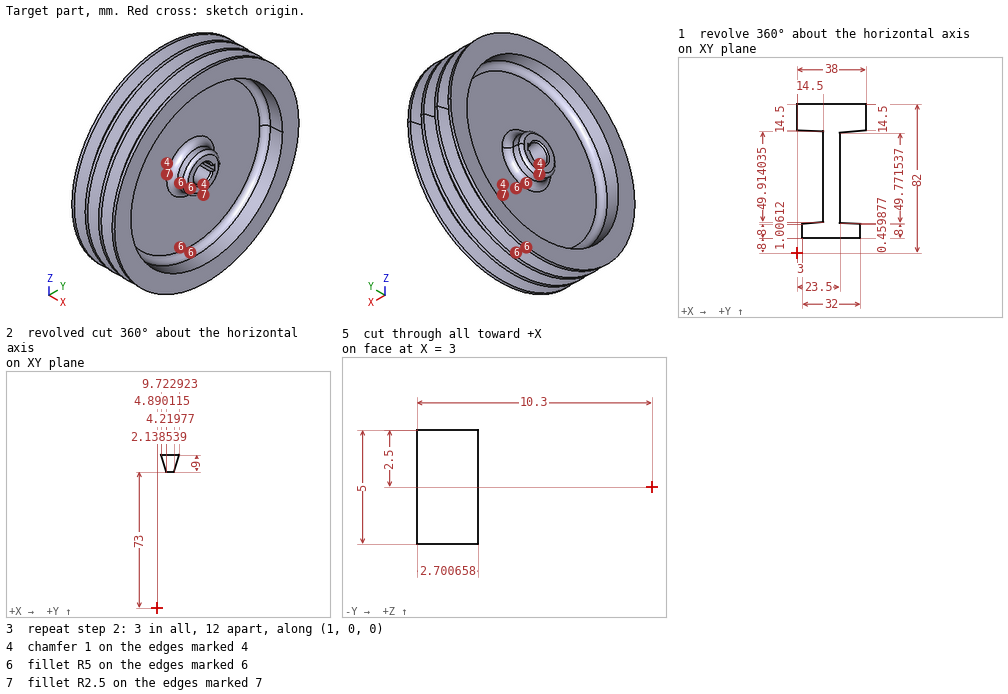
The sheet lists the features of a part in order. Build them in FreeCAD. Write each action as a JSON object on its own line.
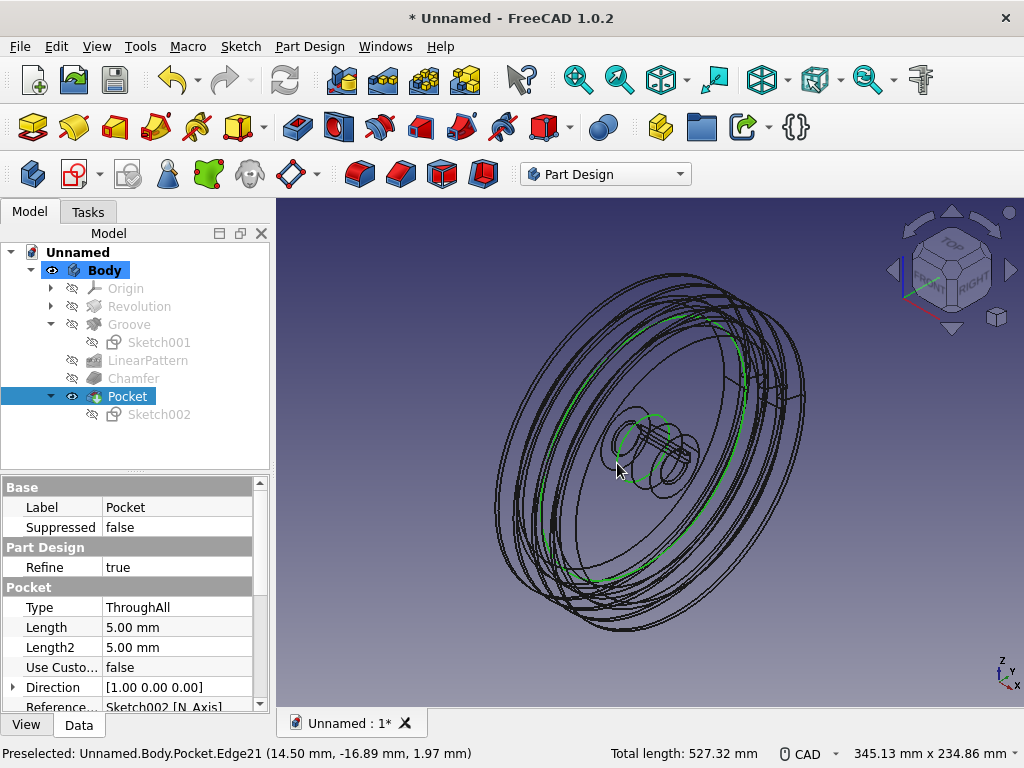
{"action": "left_click", "coordinate": [632, 470], "text": "ctrl"}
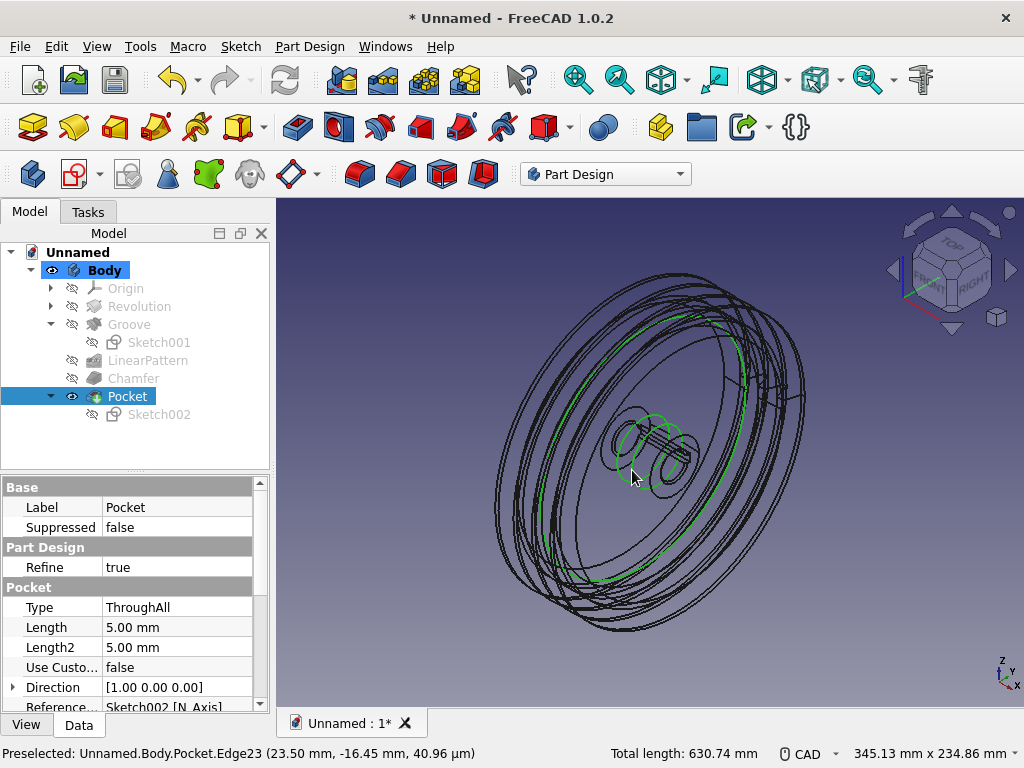
{"action": "left_click", "coordinate": [575, 572], "text": "ctrl"}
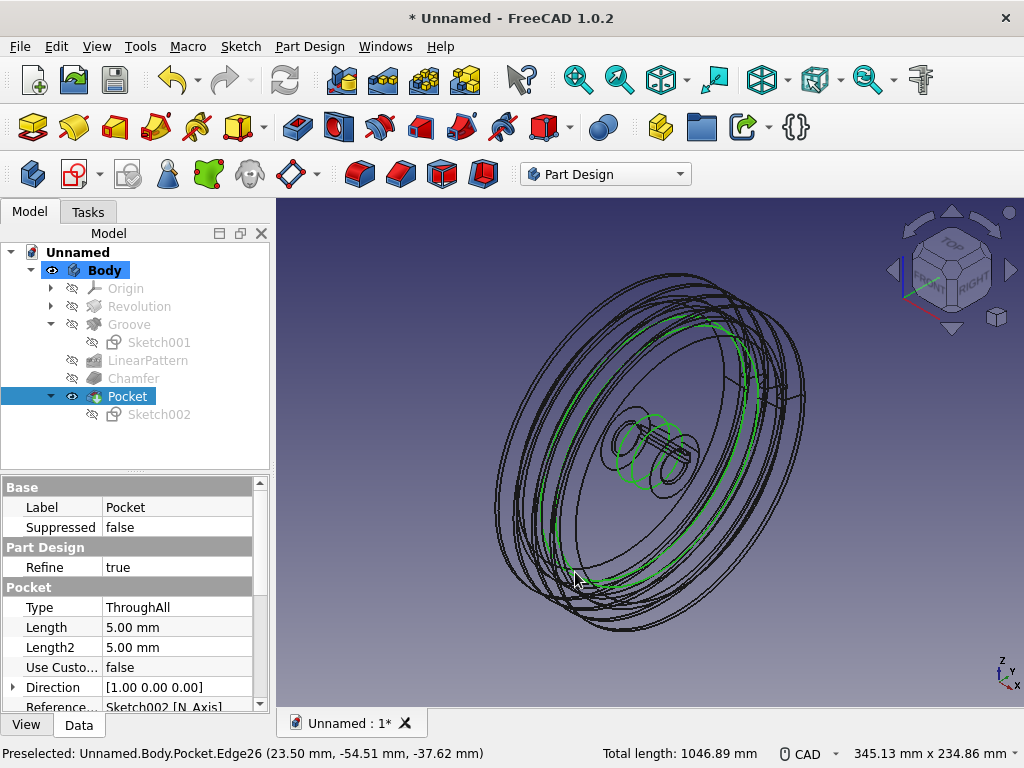
{"action": "key", "text": "v 1"}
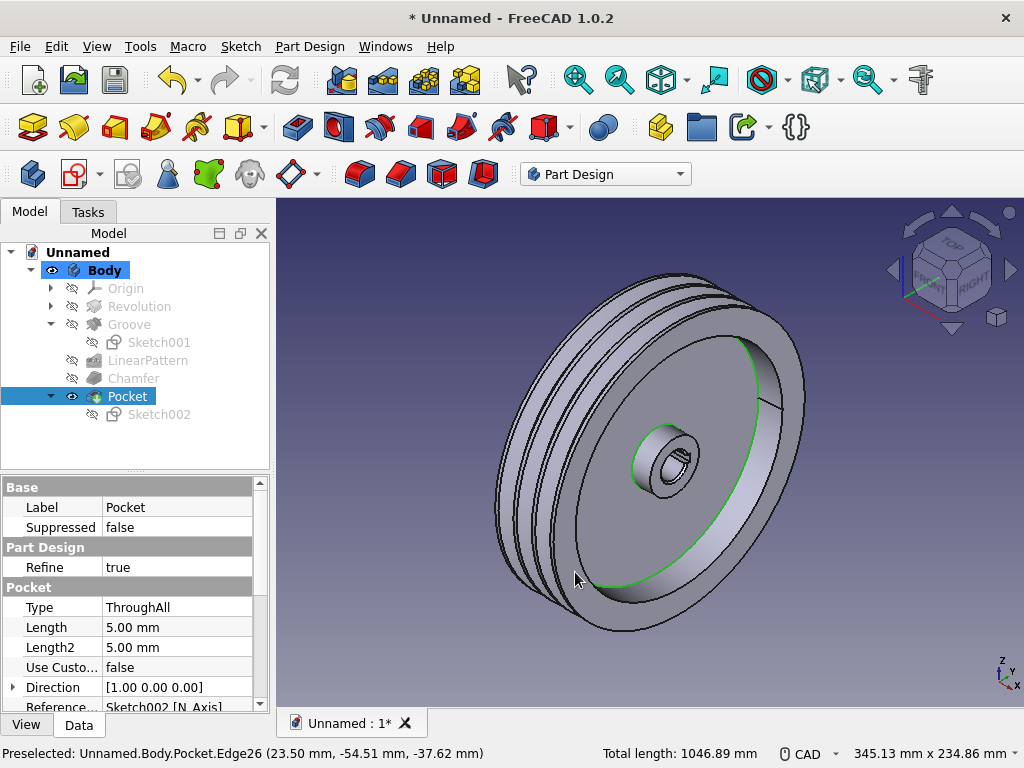
{"action": "left_click", "coordinate": [360, 174]}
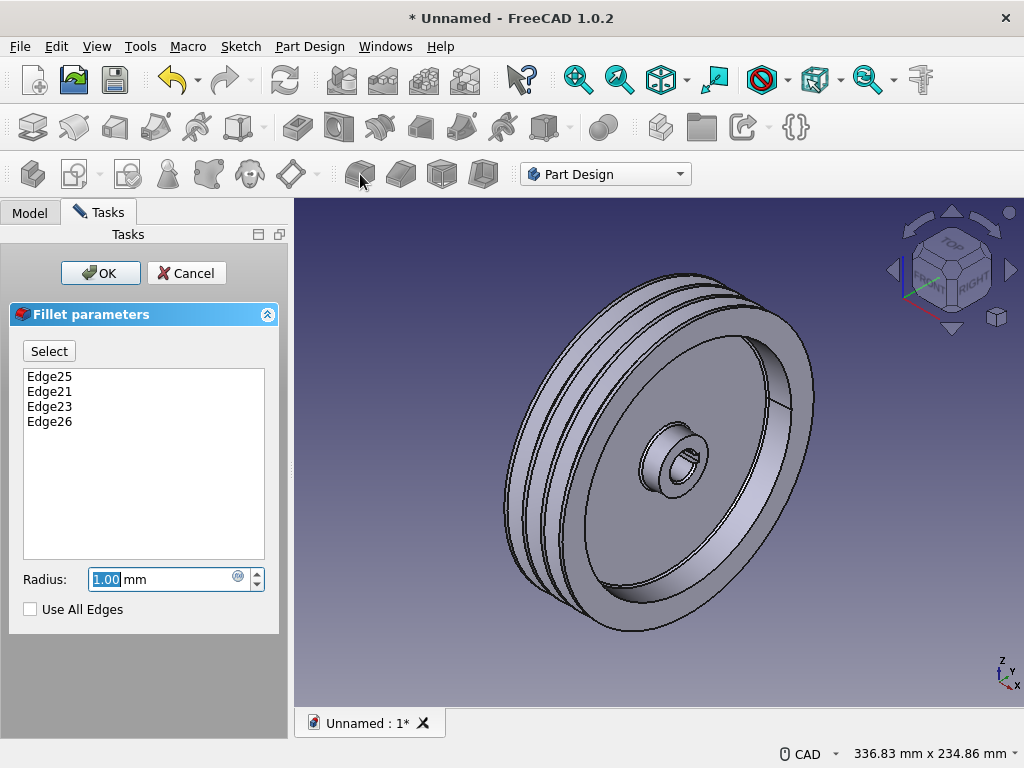
{"action": "type", "text": "5"}
{"action": "key", "text": "Tab"}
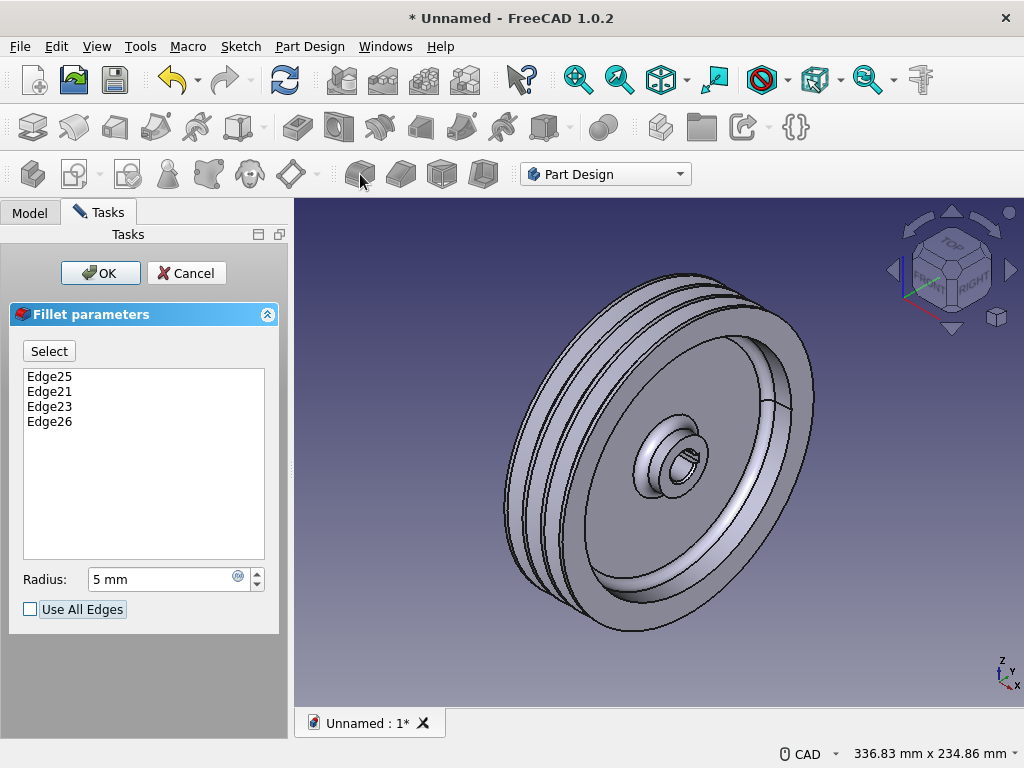
{"action": "left_click", "coordinate": [101, 273]}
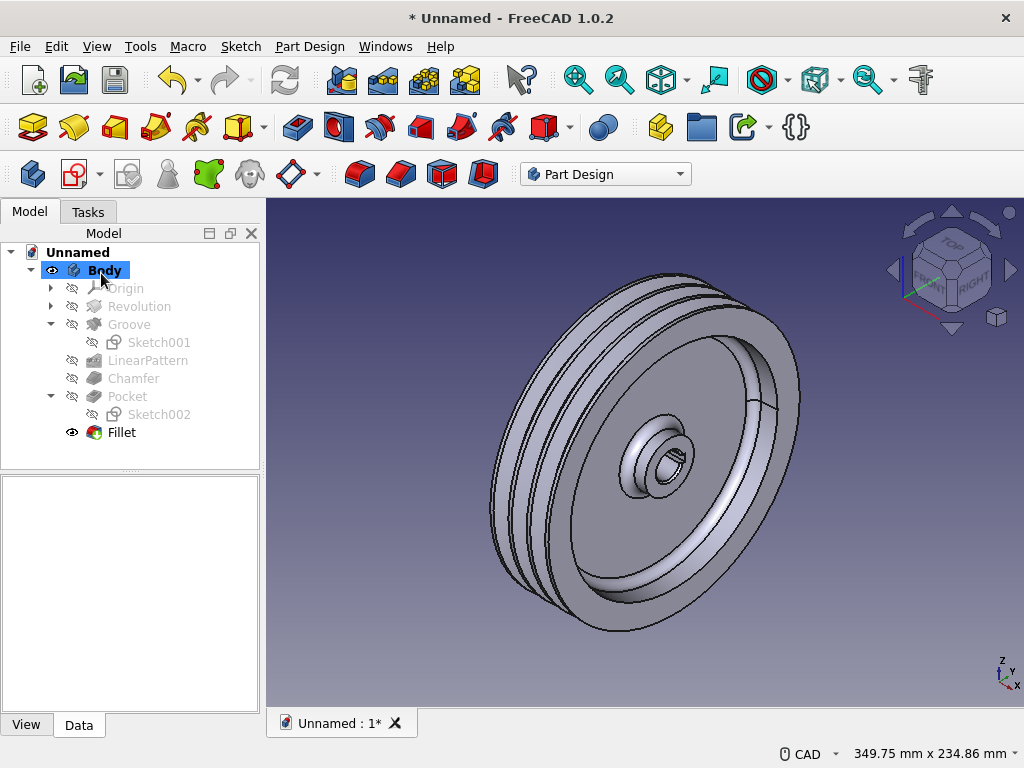
{"action": "left_click", "coordinate": [645, 480]}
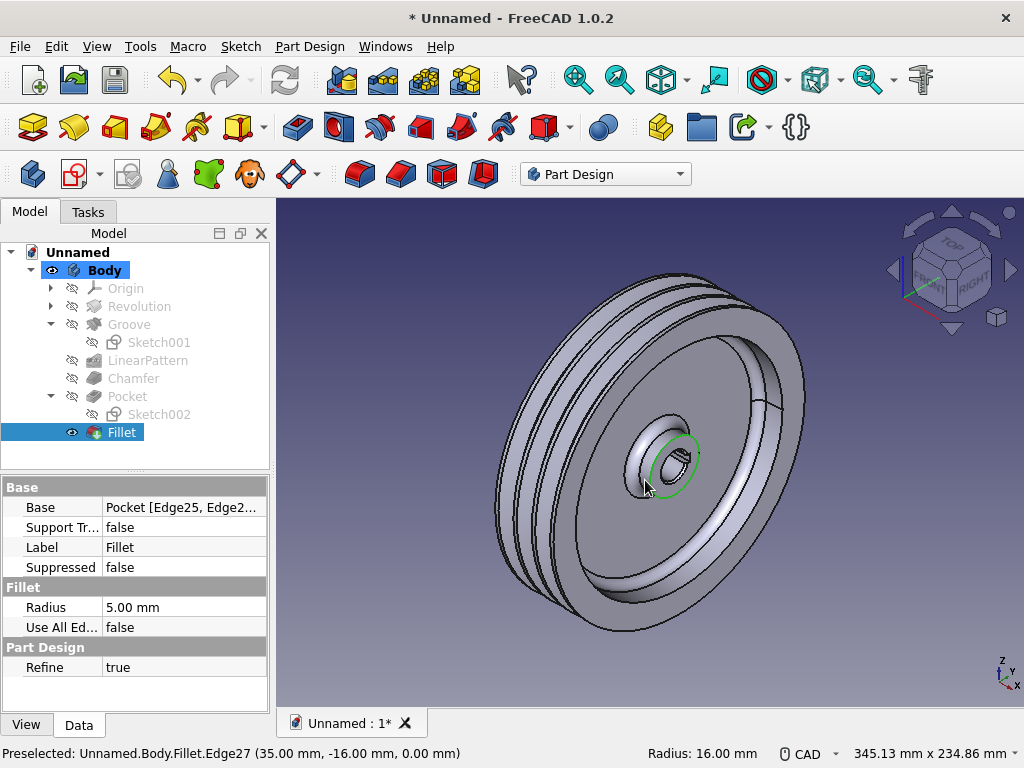
{"action": "key", "text": "2"}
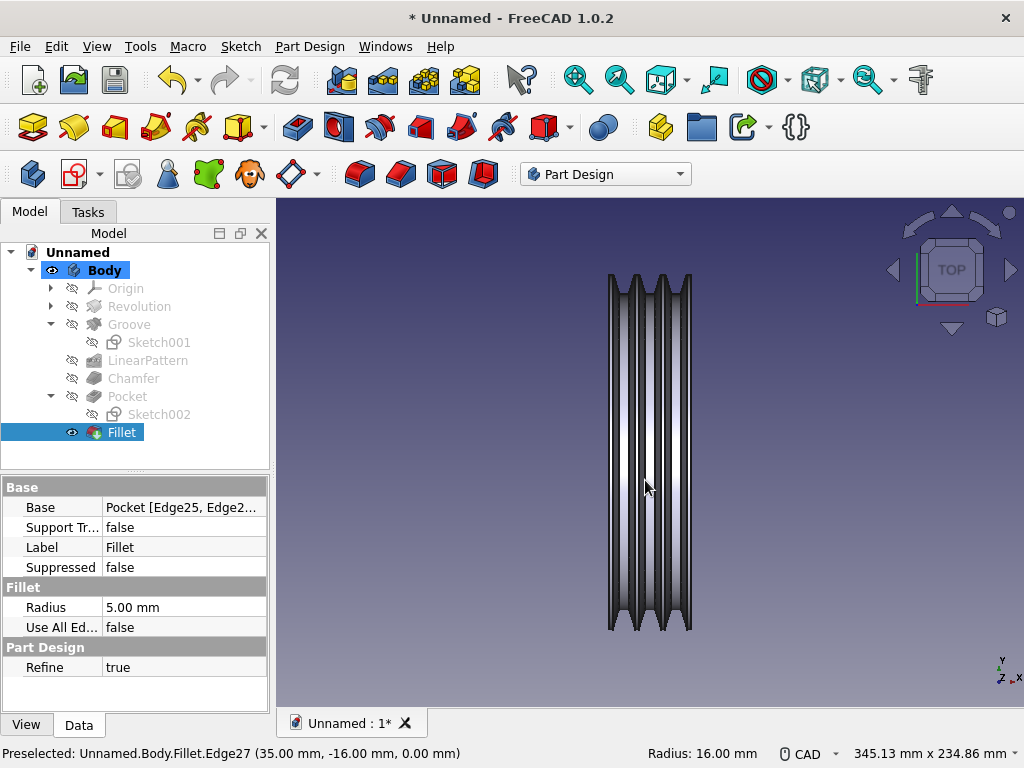
{"action": "key", "text": "0"}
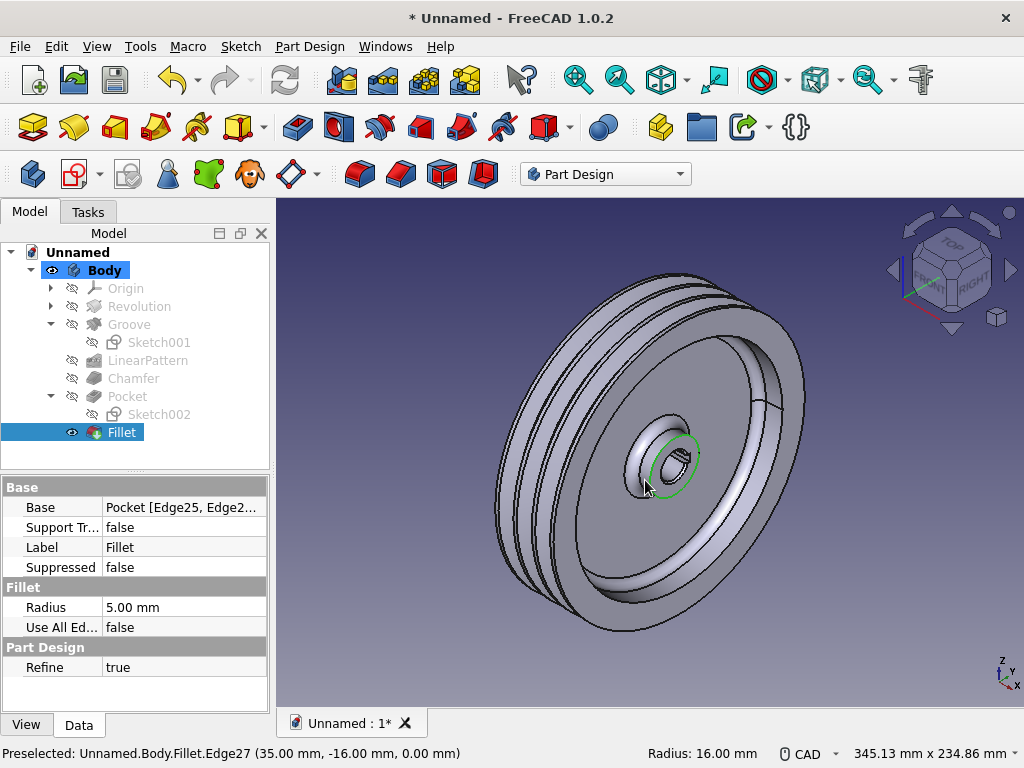
{"action": "key", "text": "1"}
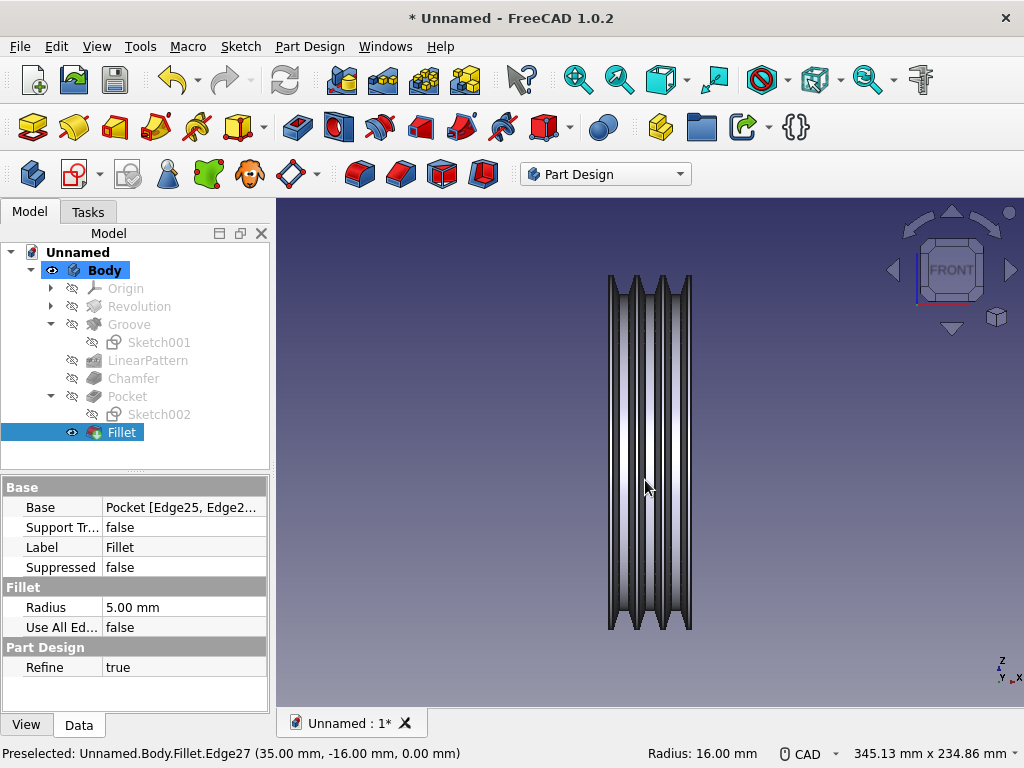
{"action": "key", "text": "3"}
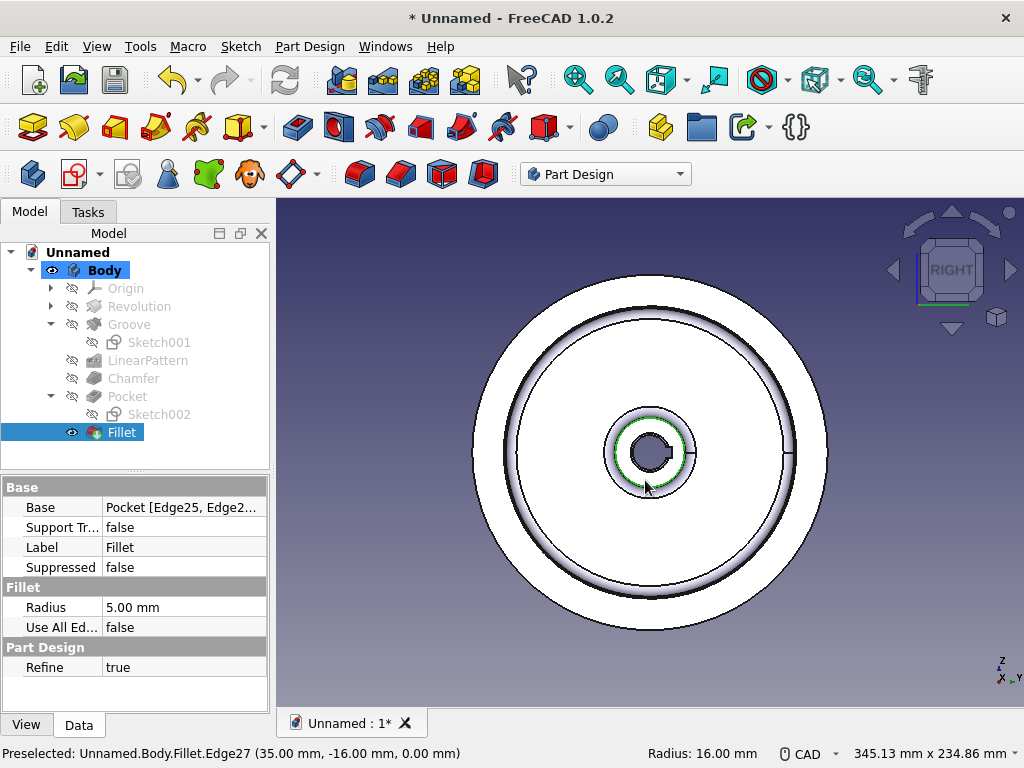
{"action": "key", "text": "5"}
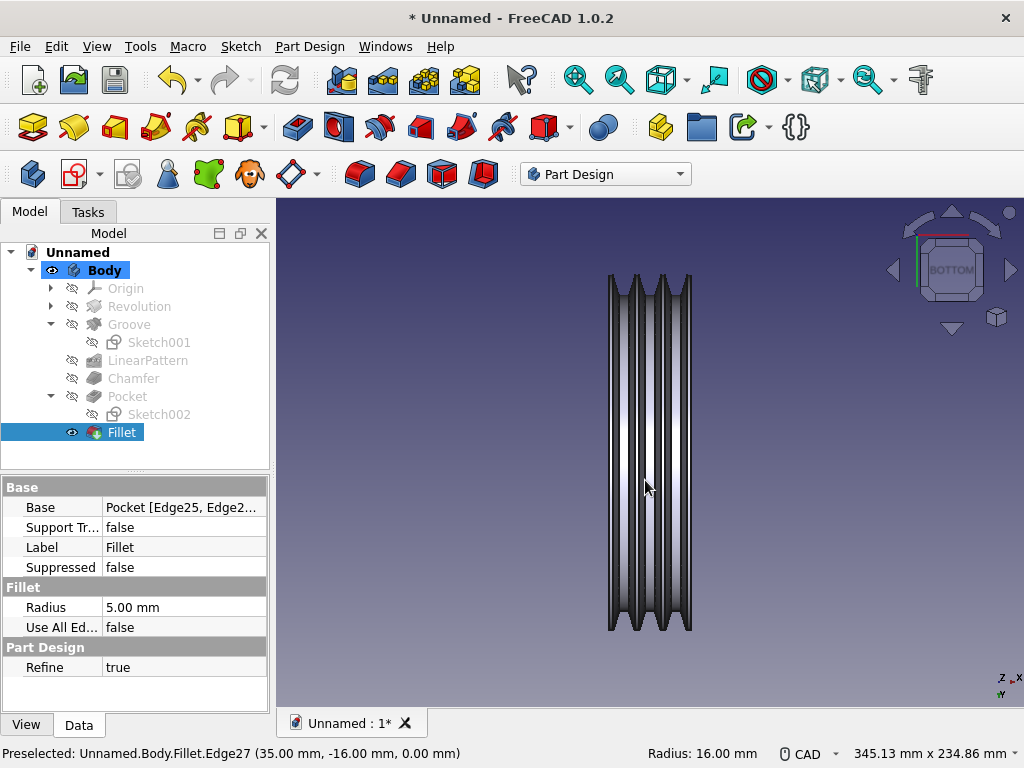
{"action": "key", "text": "4"}